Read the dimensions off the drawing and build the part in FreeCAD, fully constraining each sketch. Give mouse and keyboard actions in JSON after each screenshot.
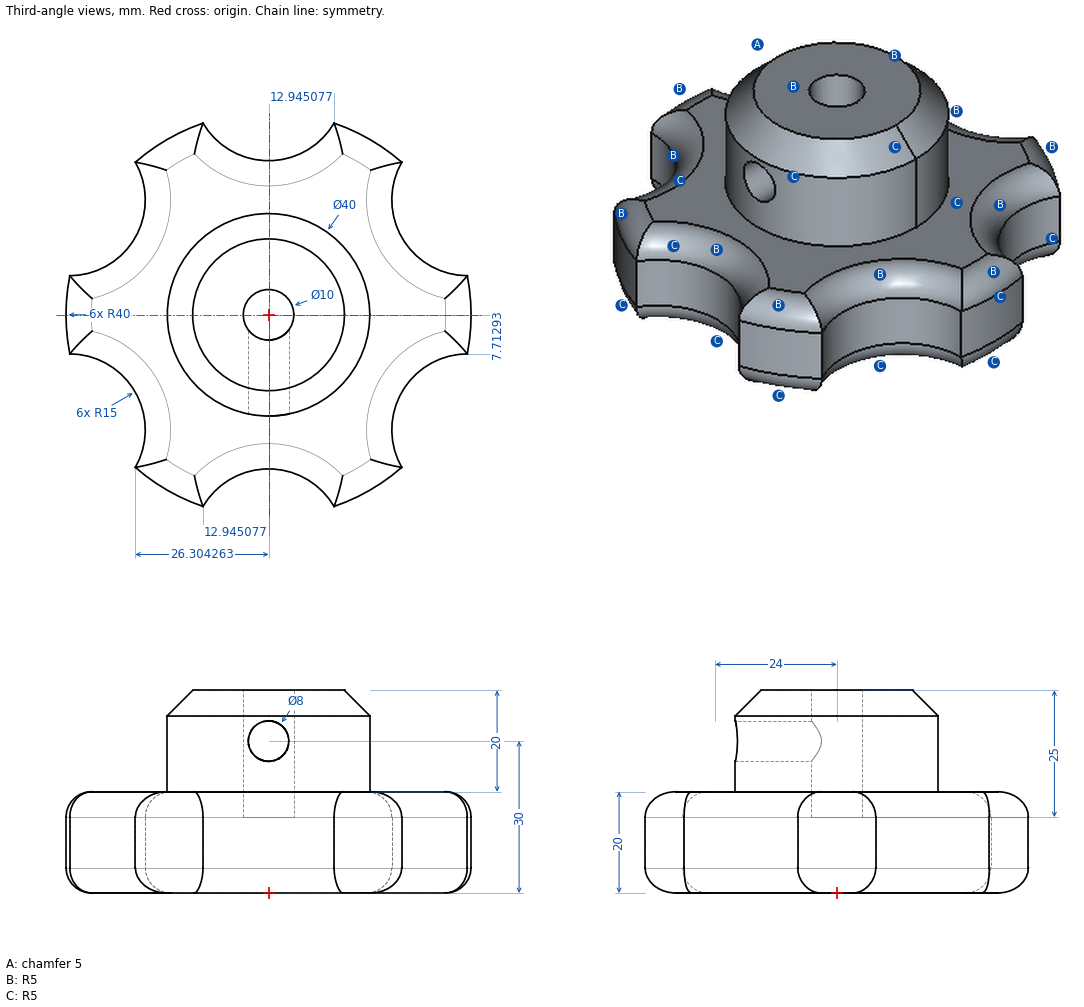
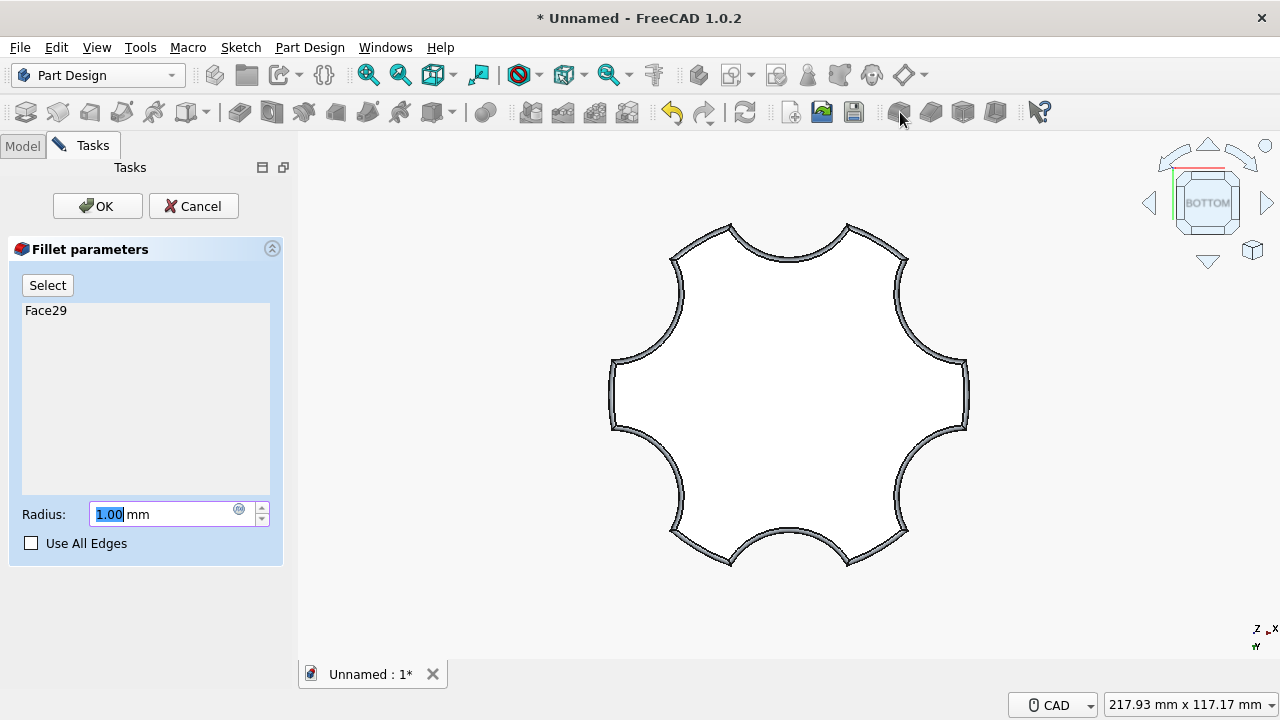
{"action": "type", "text": "5"}
{"action": "key", "text": "Tab"}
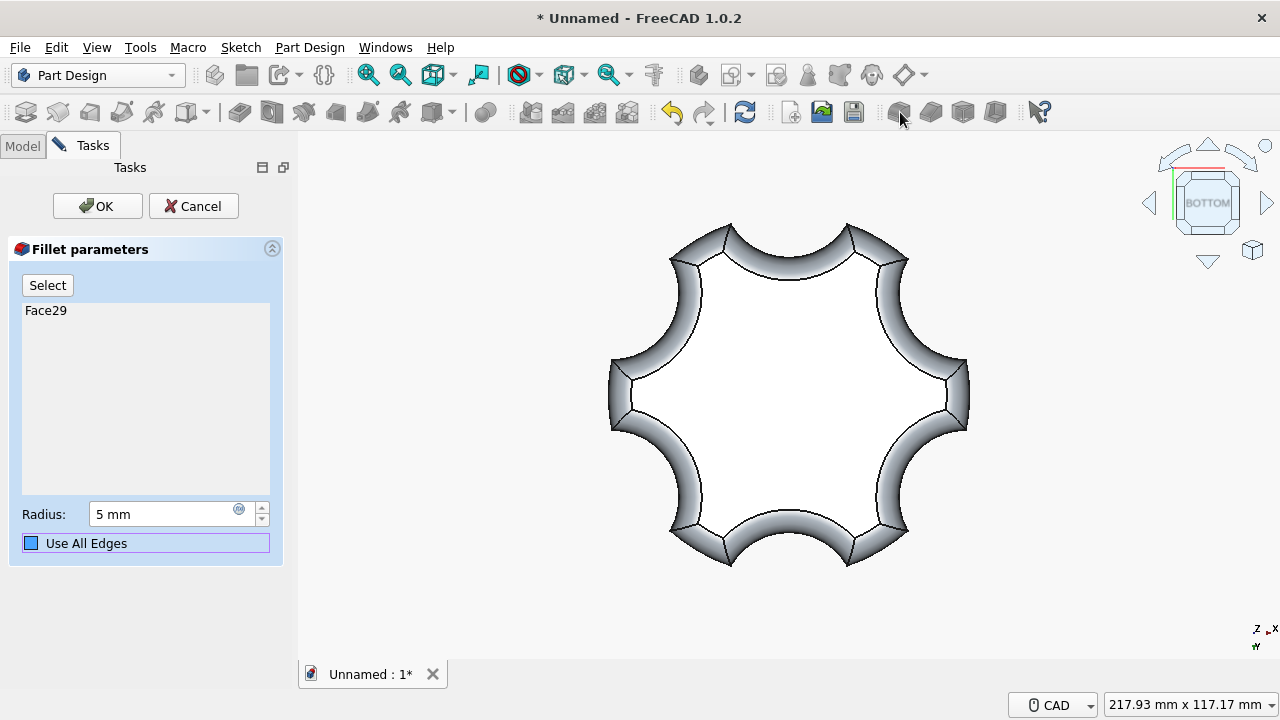
{"action": "left_click", "coordinate": [98, 206]}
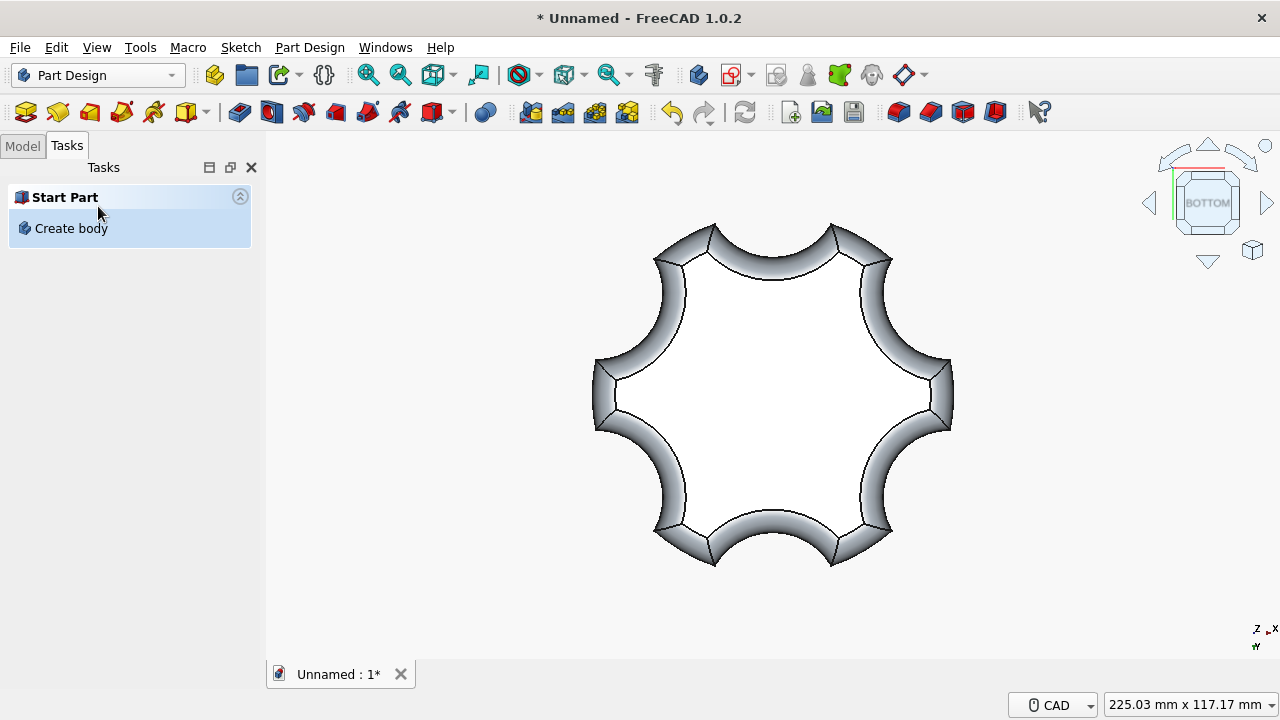
{"action": "key", "text": "0"}